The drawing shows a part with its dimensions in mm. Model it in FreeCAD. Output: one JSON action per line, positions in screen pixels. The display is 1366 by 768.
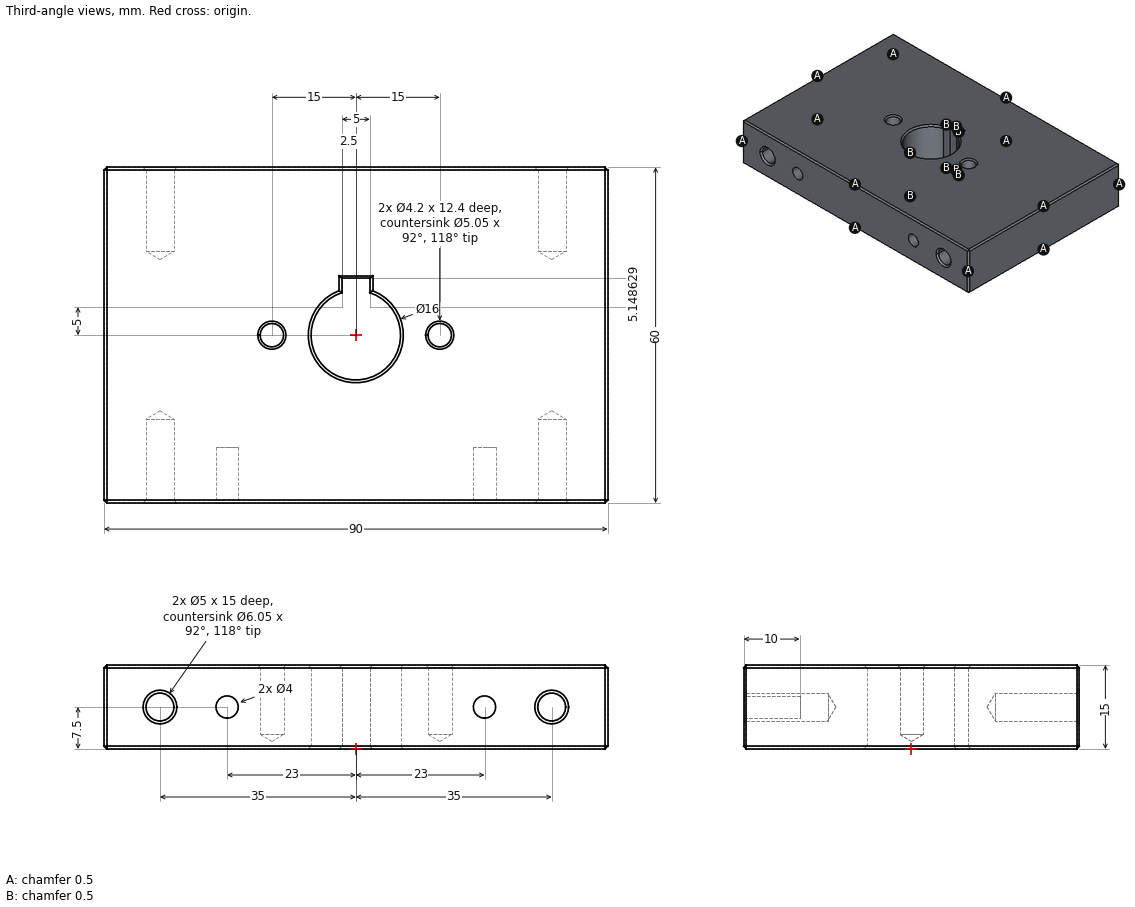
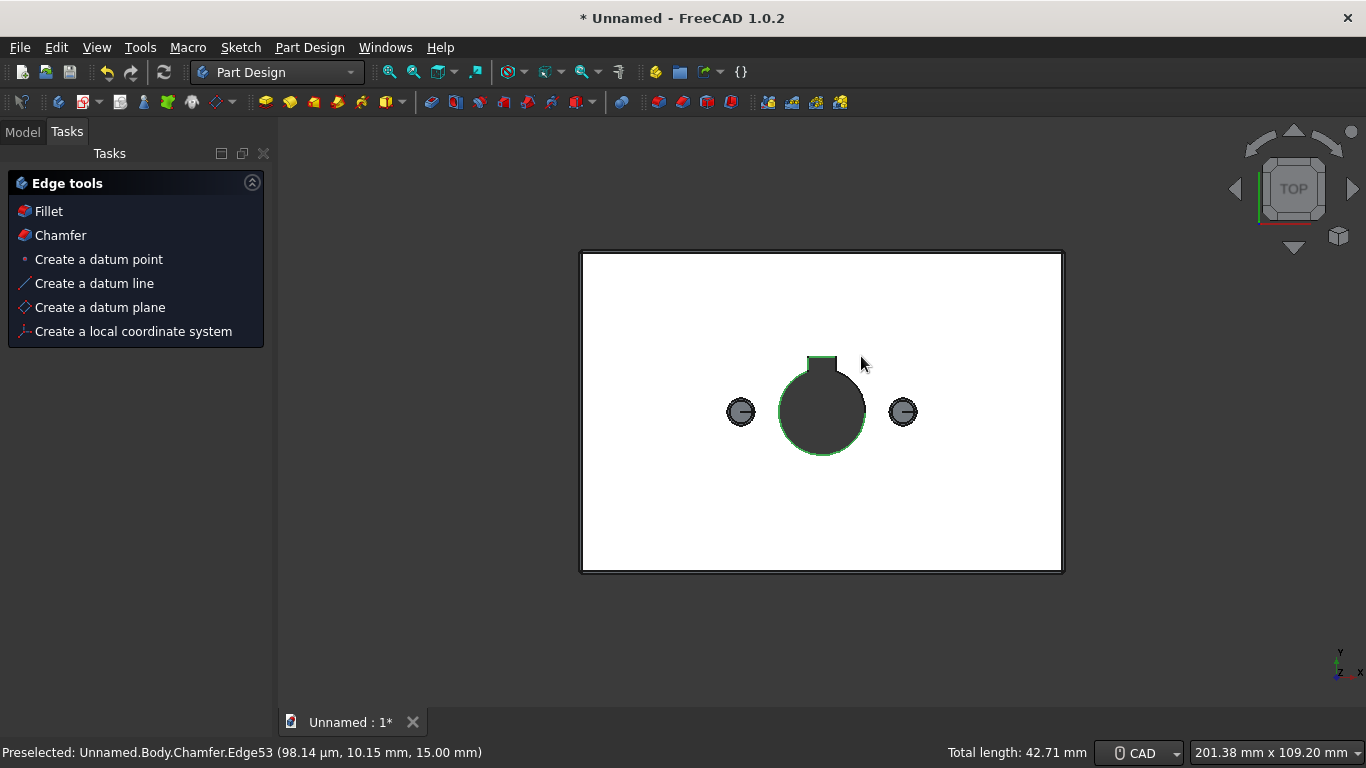
{"action": "left_click", "coordinate": [836, 363], "text": "ctrl"}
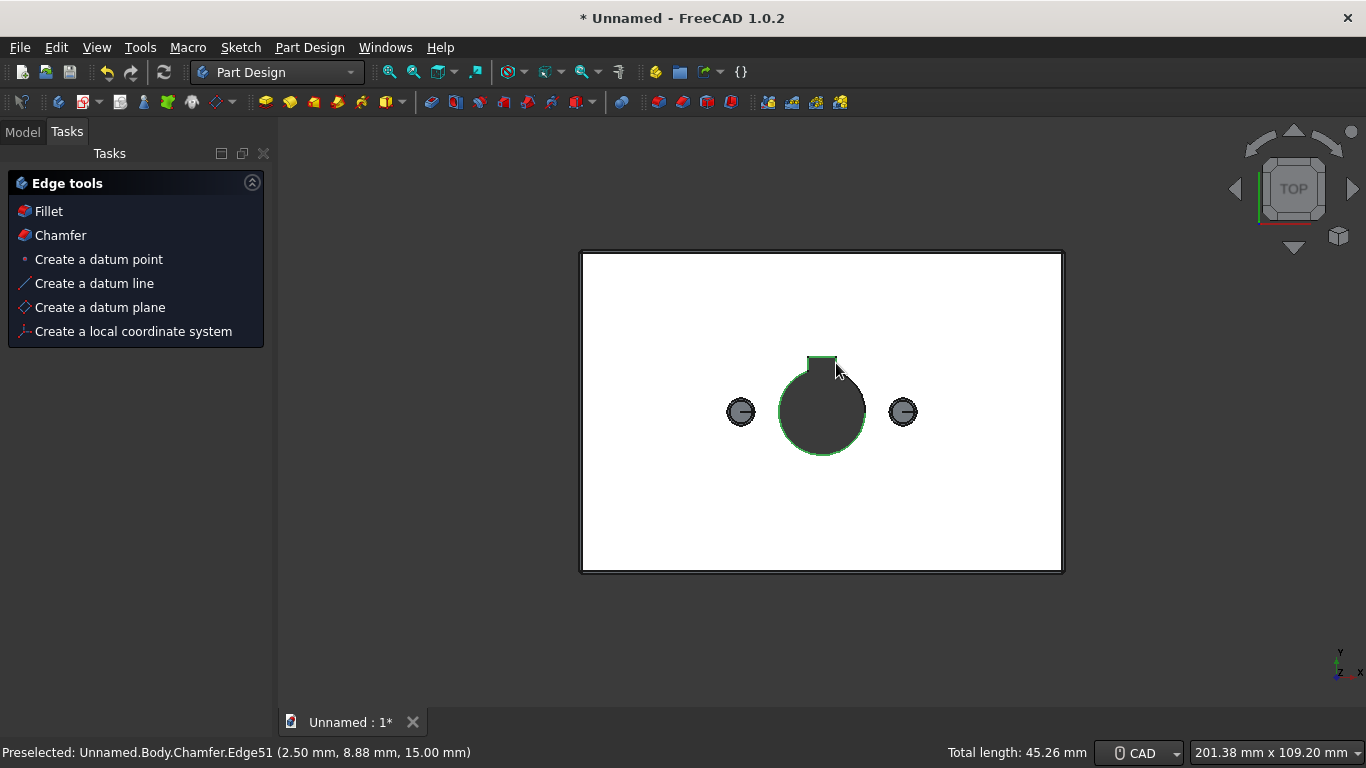
{"action": "key", "text": "1"}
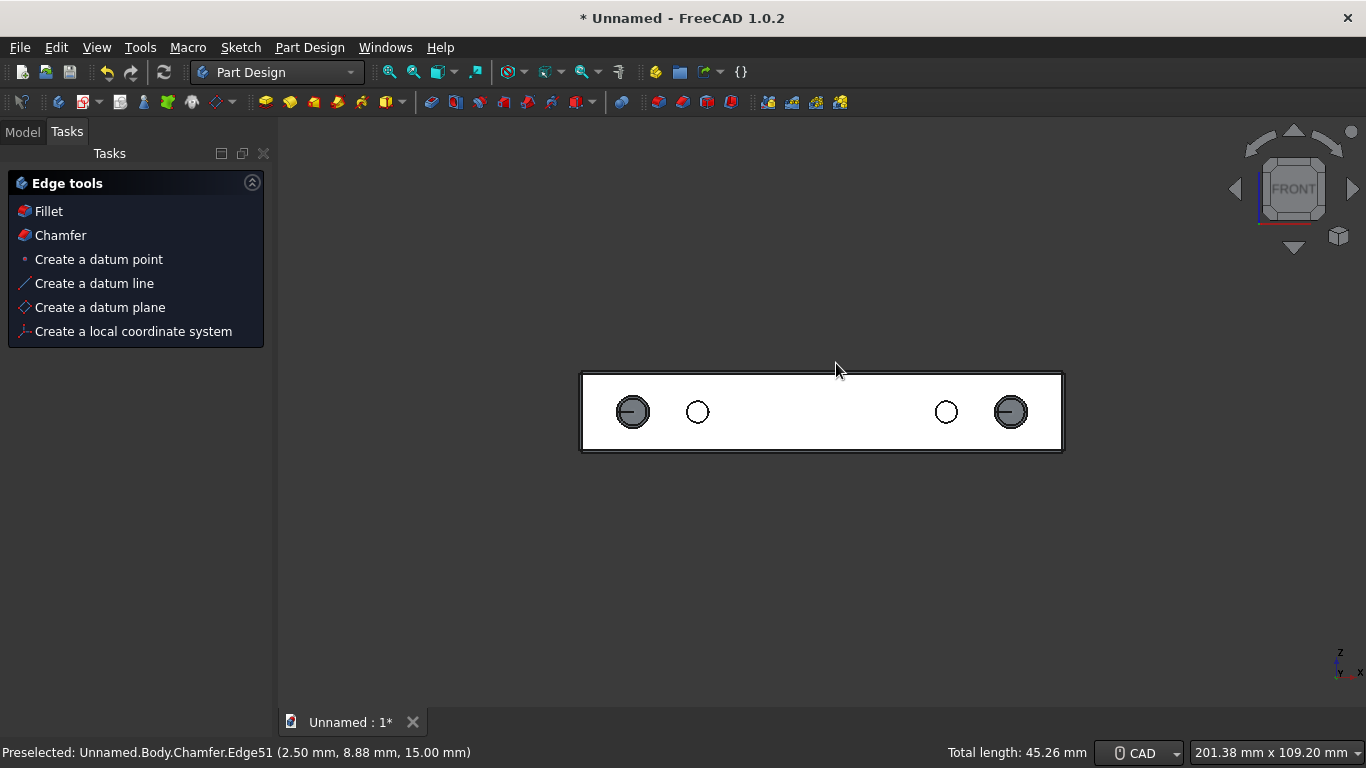
{"action": "key", "text": "v f"}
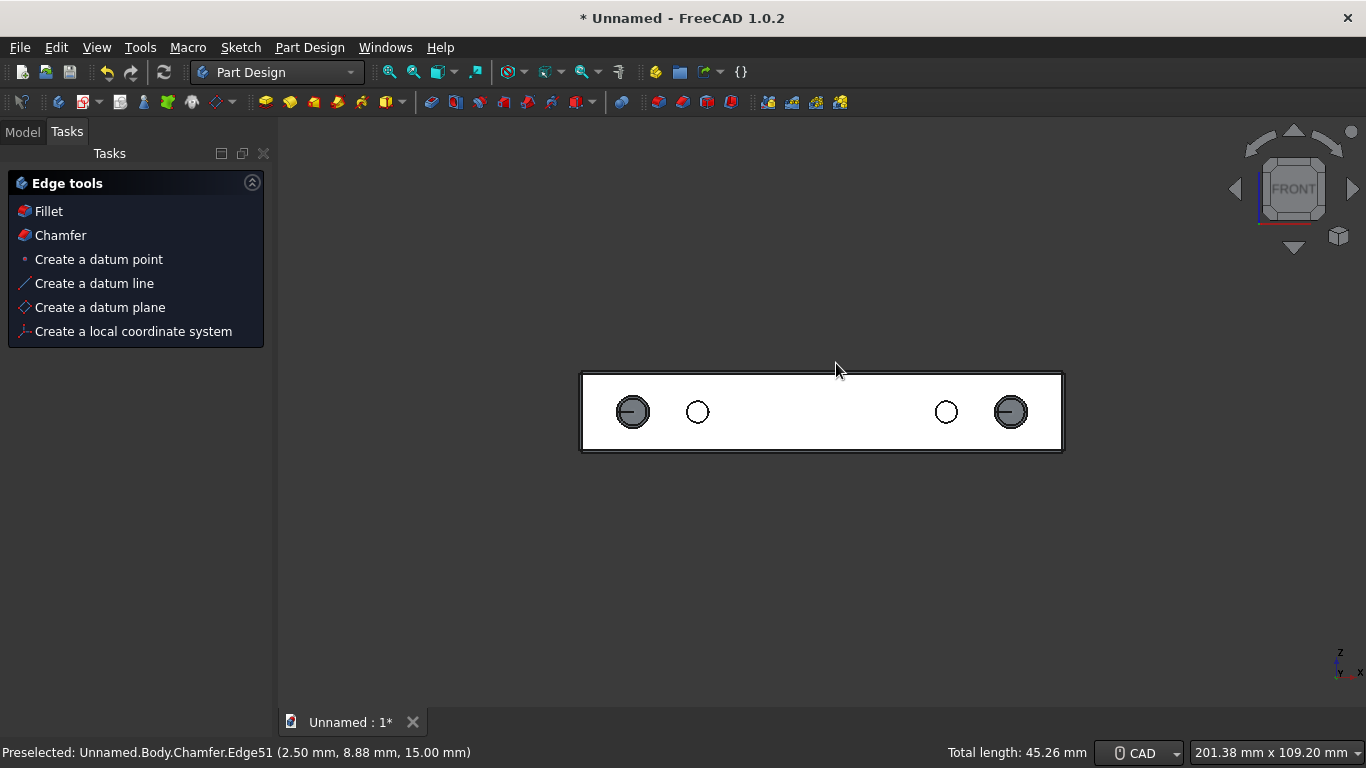
{"action": "key", "text": "3"}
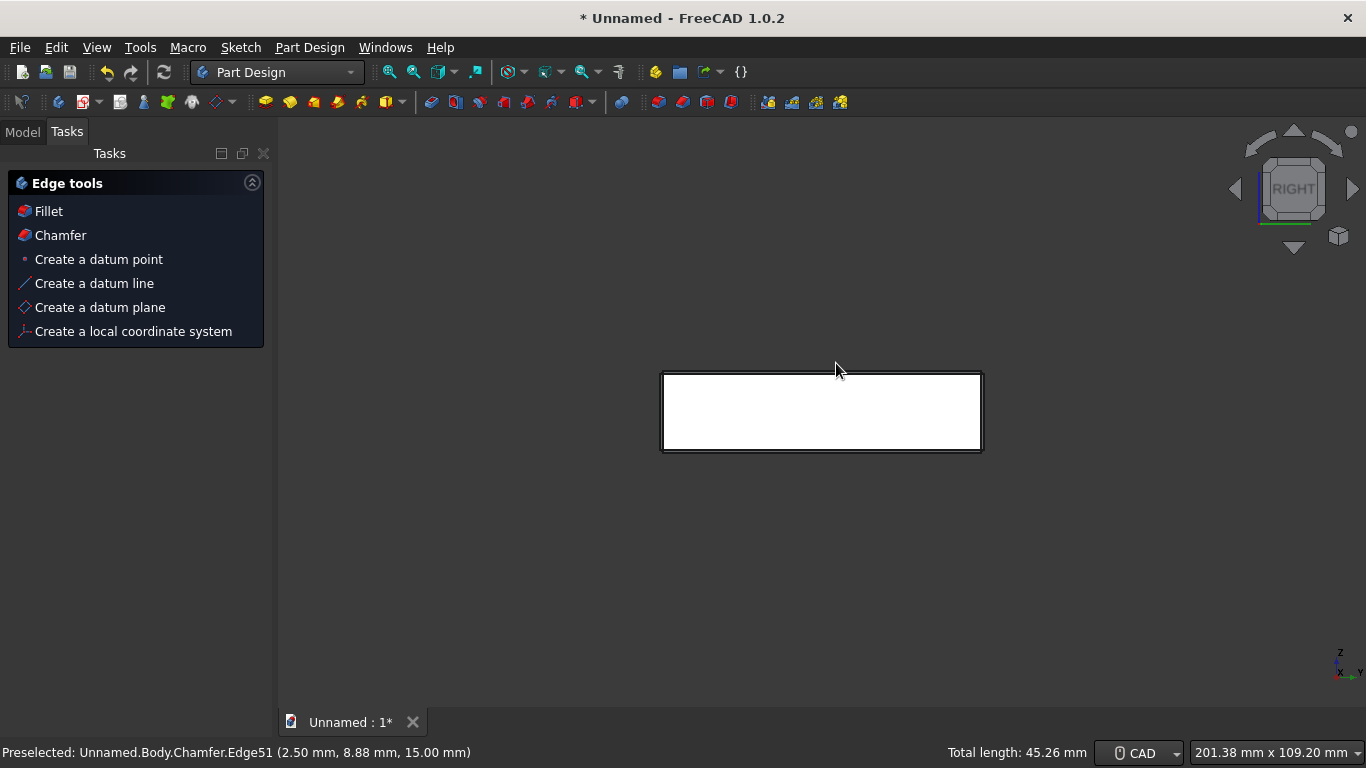
{"action": "key", "text": "v f"}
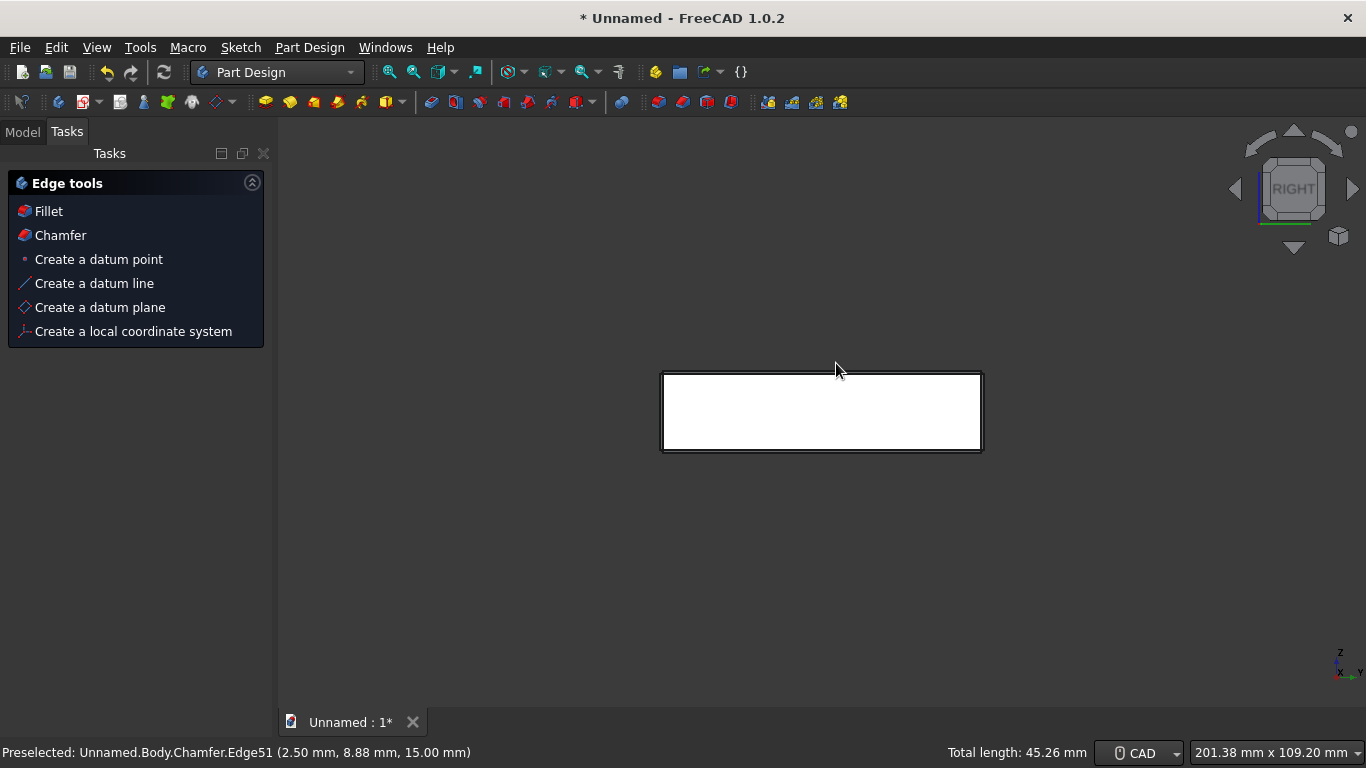
{"action": "key", "text": "5"}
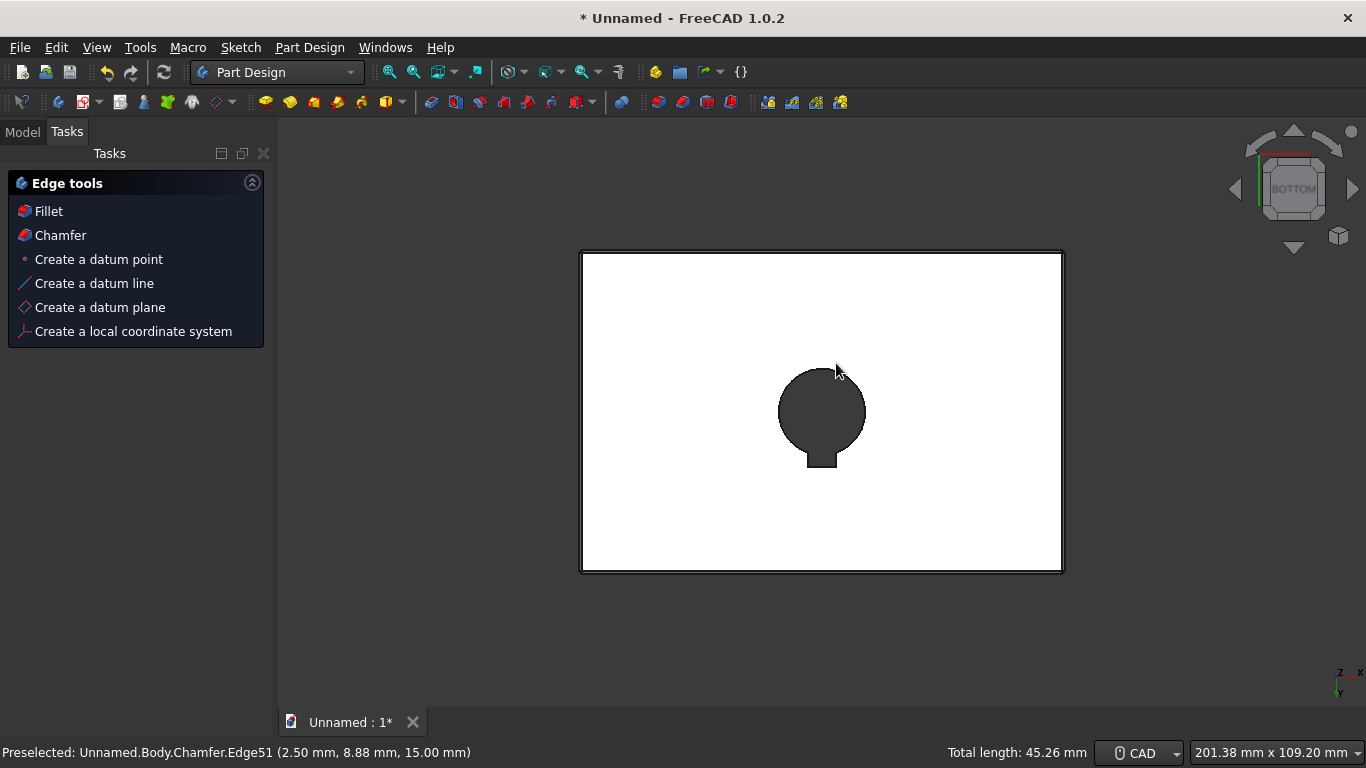
{"action": "left_click", "coordinate": [808, 459], "text": "ctrl"}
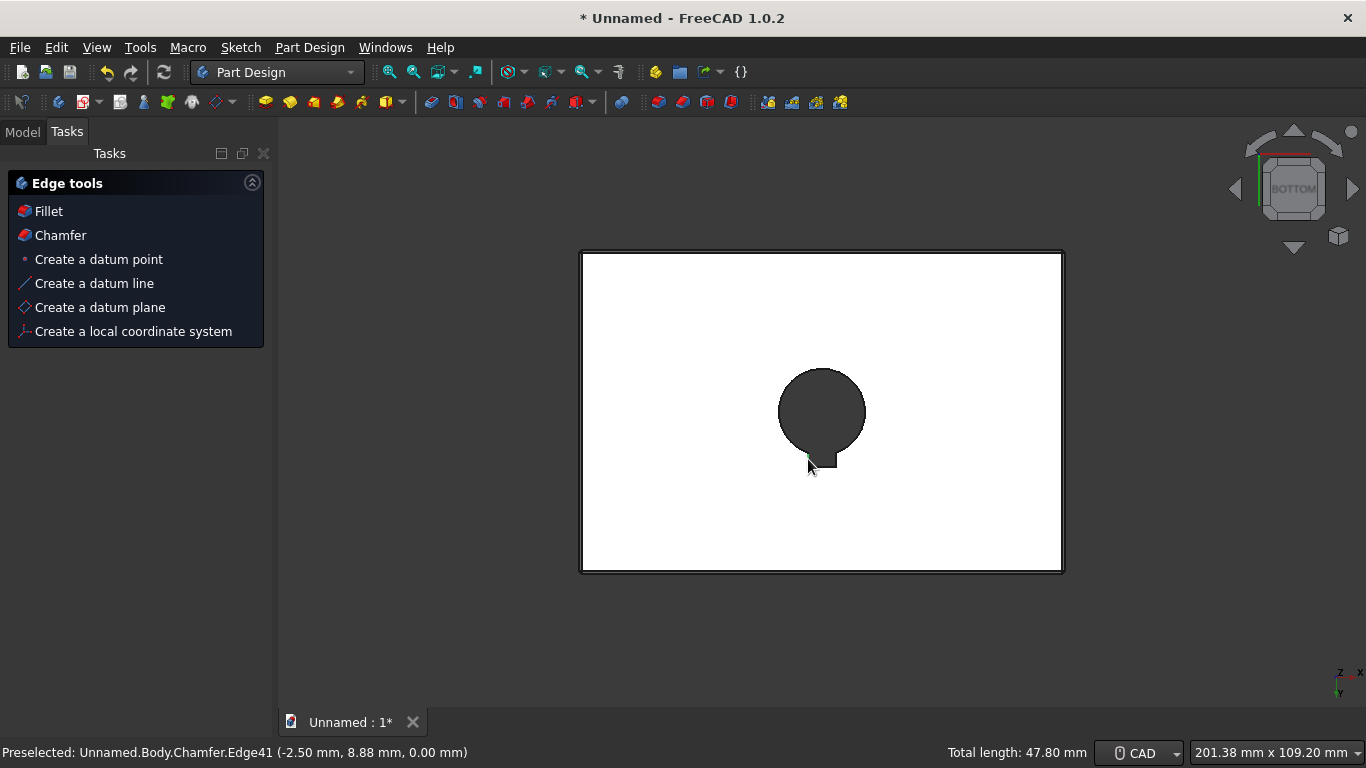
{"action": "left_click", "coordinate": [836, 459], "text": "ctrl"}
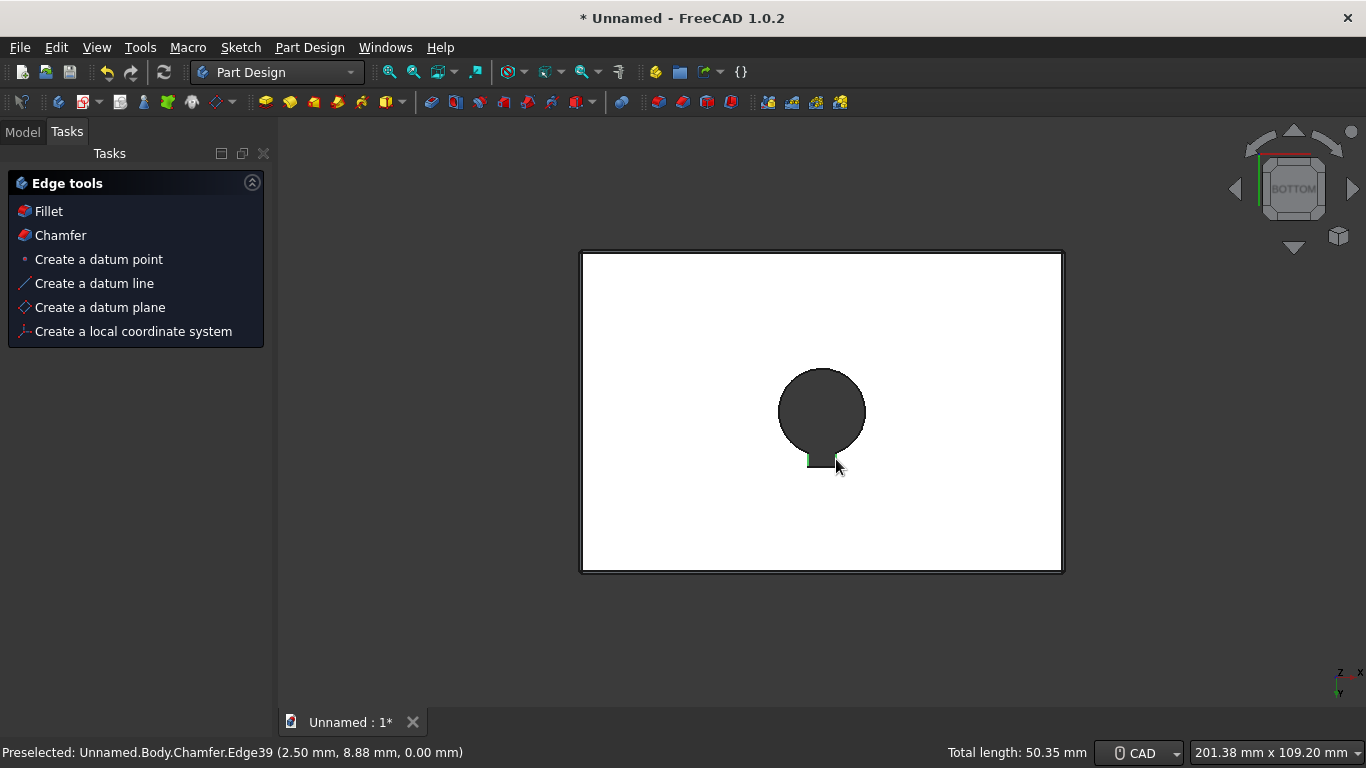
{"action": "key", "text": "4"}